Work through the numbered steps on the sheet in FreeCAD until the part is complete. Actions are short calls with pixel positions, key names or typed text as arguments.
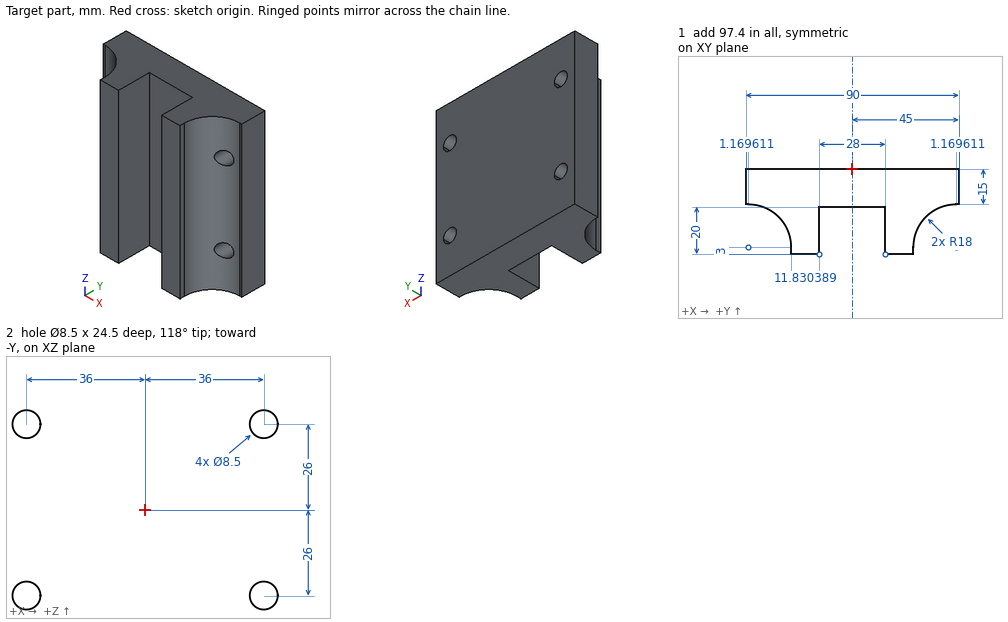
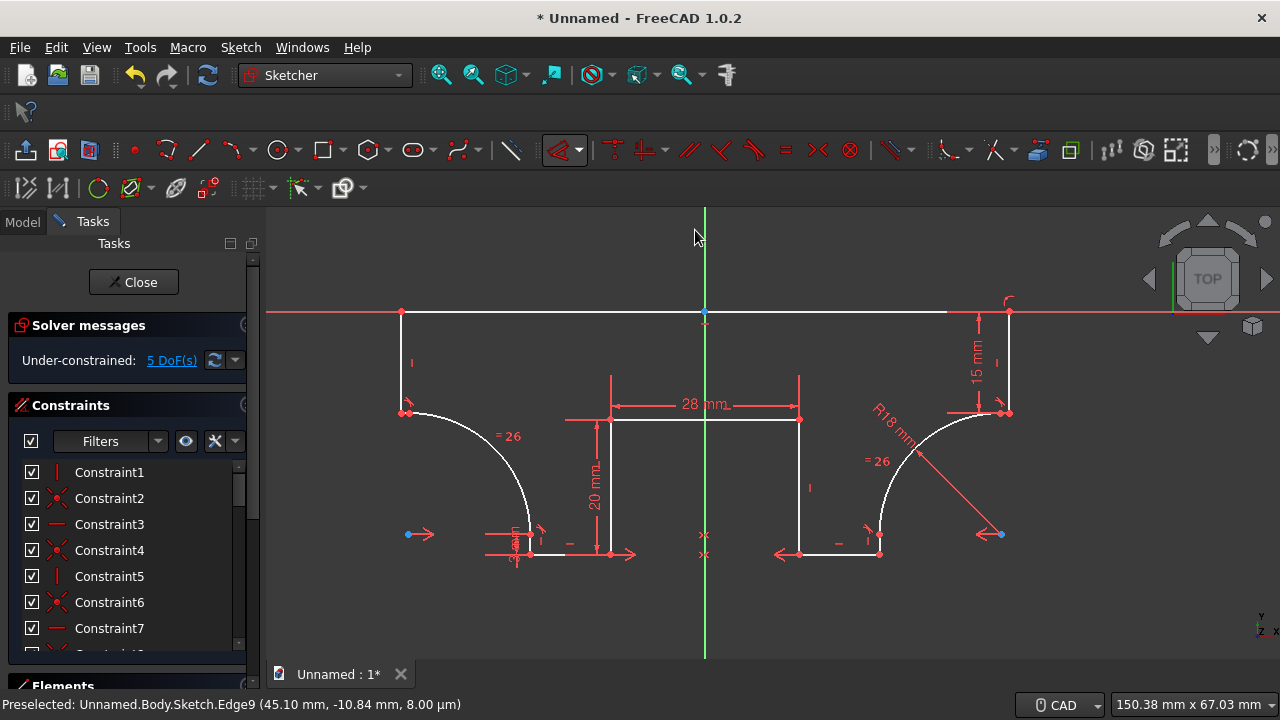
click(827, 312)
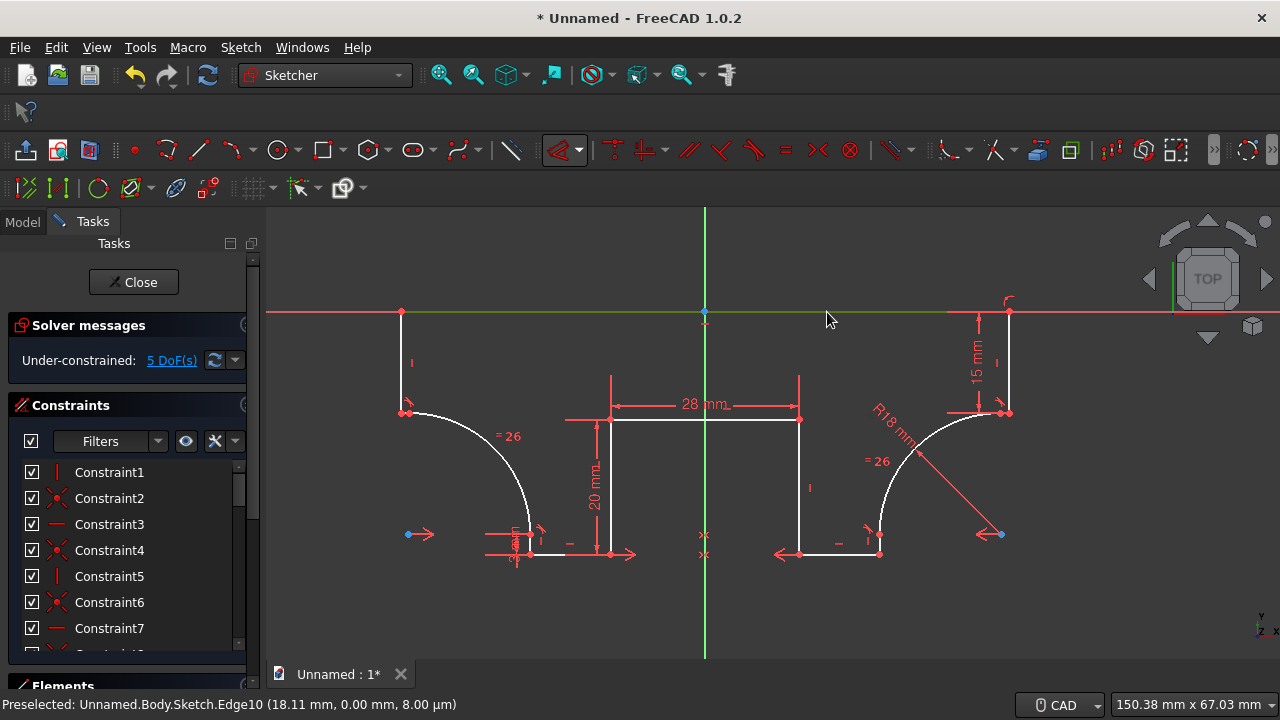
click(582, 150)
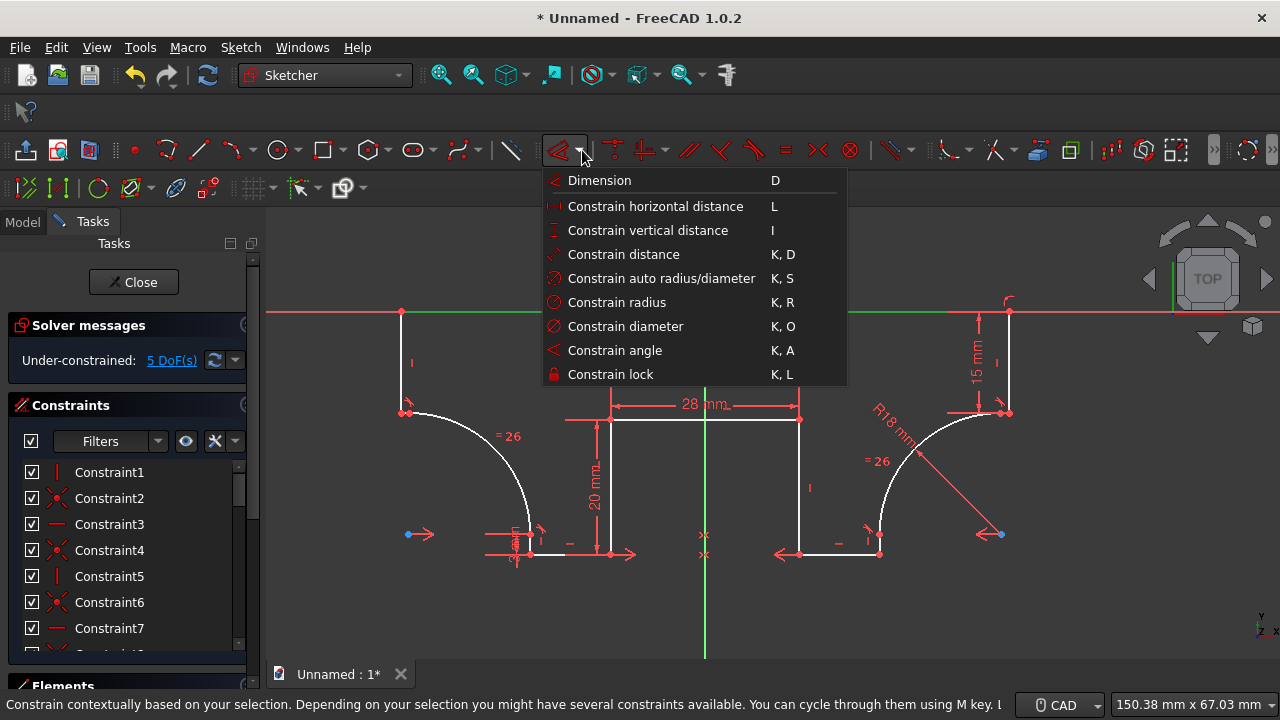
click(695, 206)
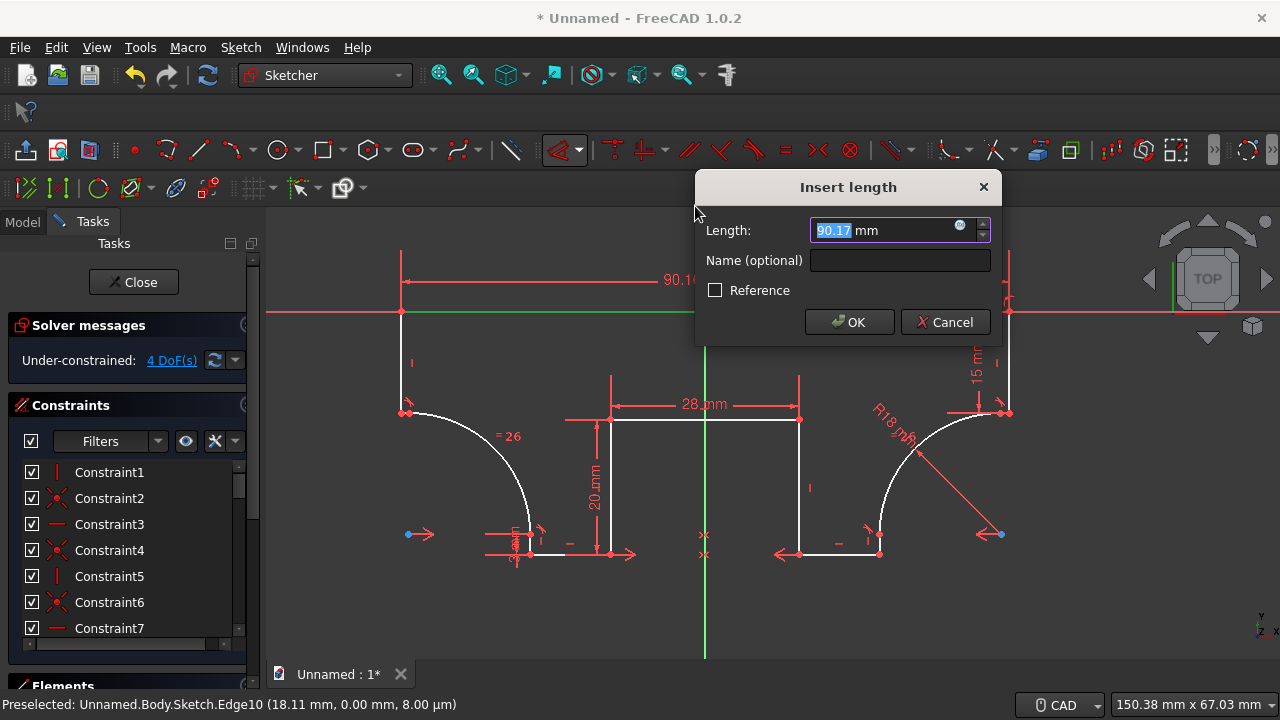
text(90)
key(Return)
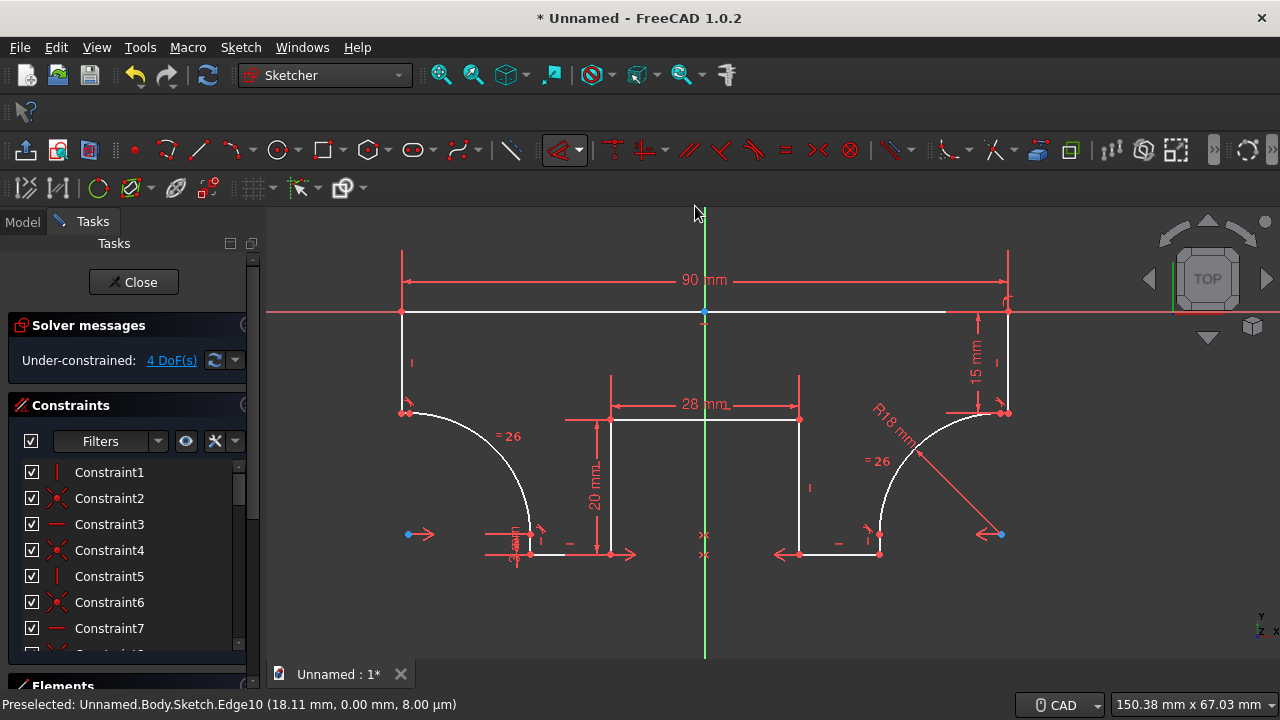
scroll(1008, 413, up, 3)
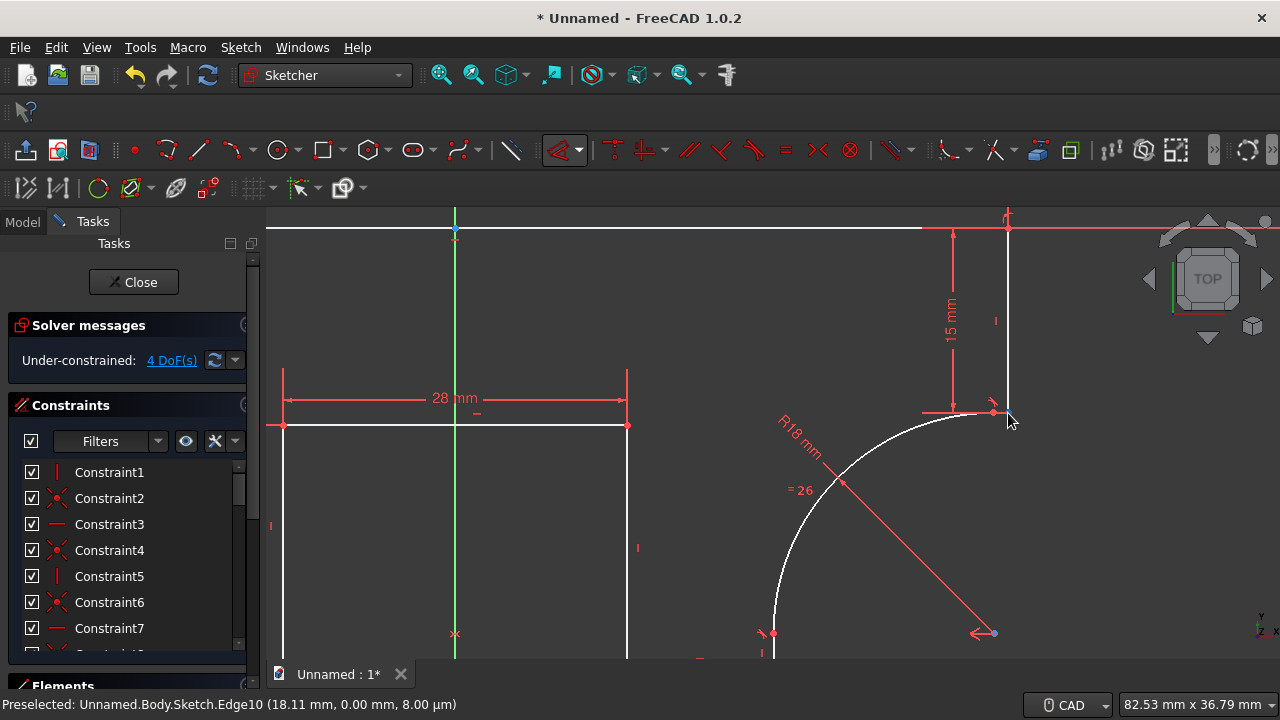
click(1008, 413)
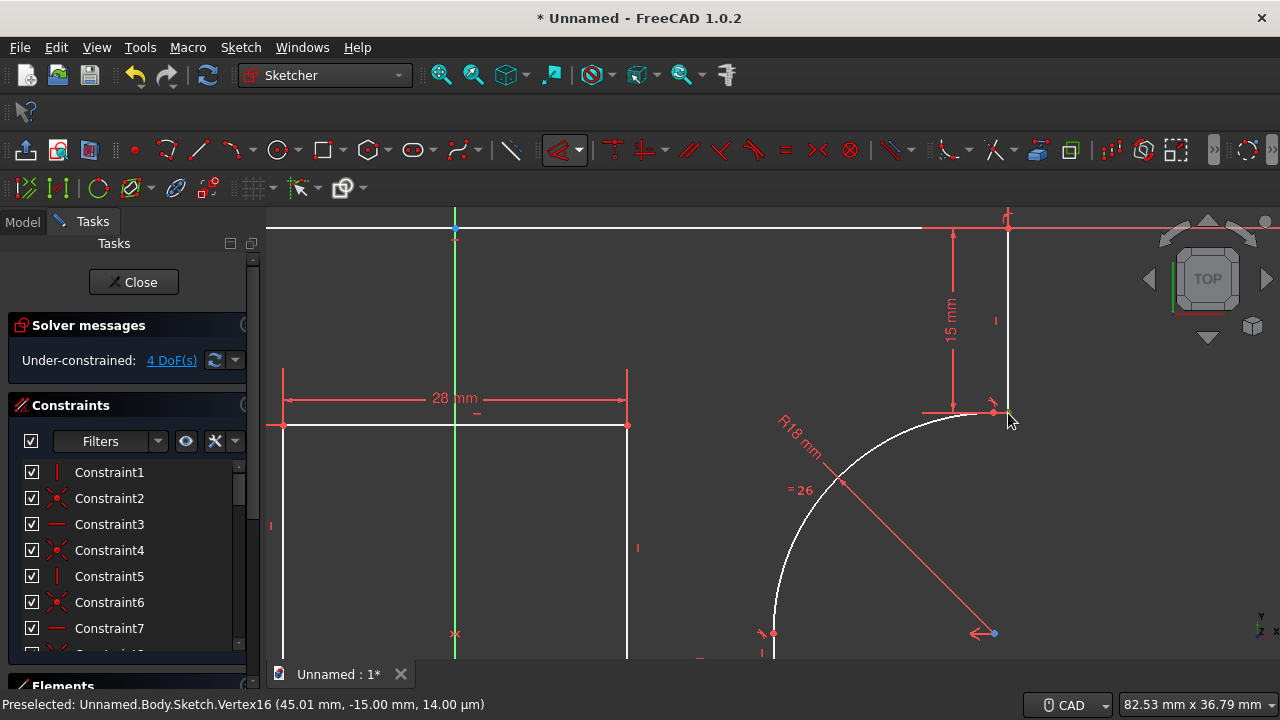
click(582, 150)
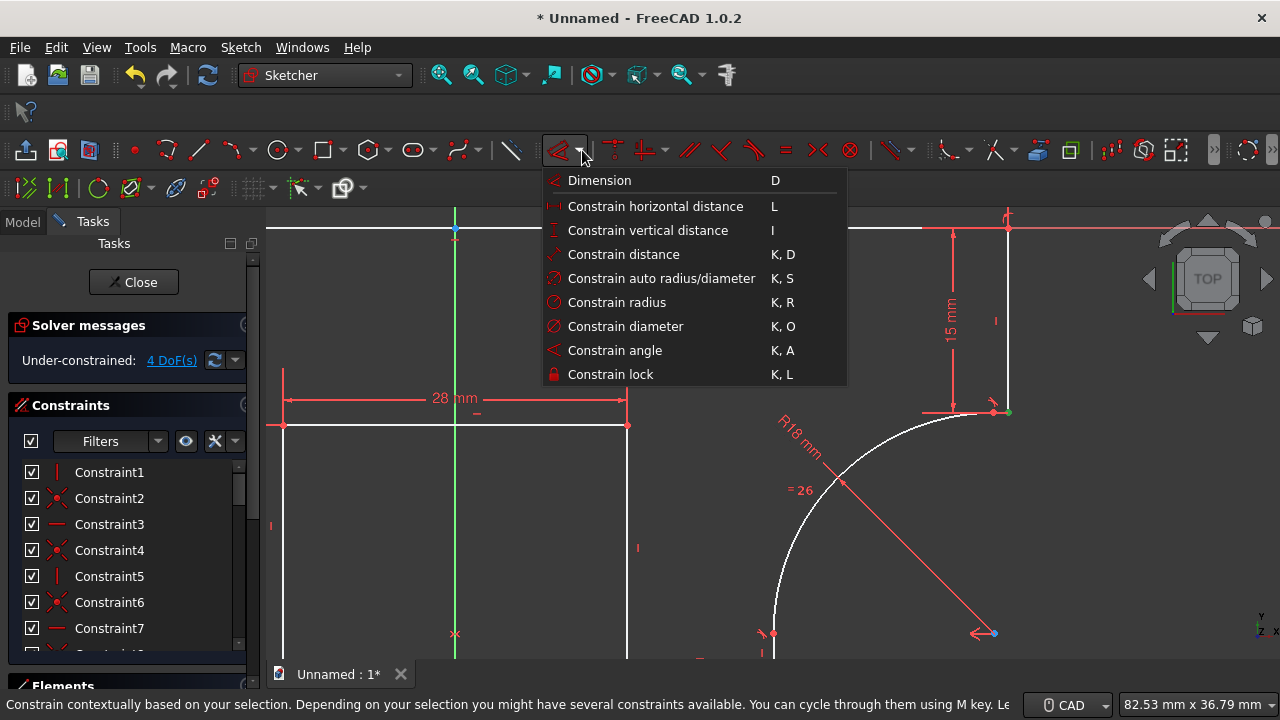
click(695, 206)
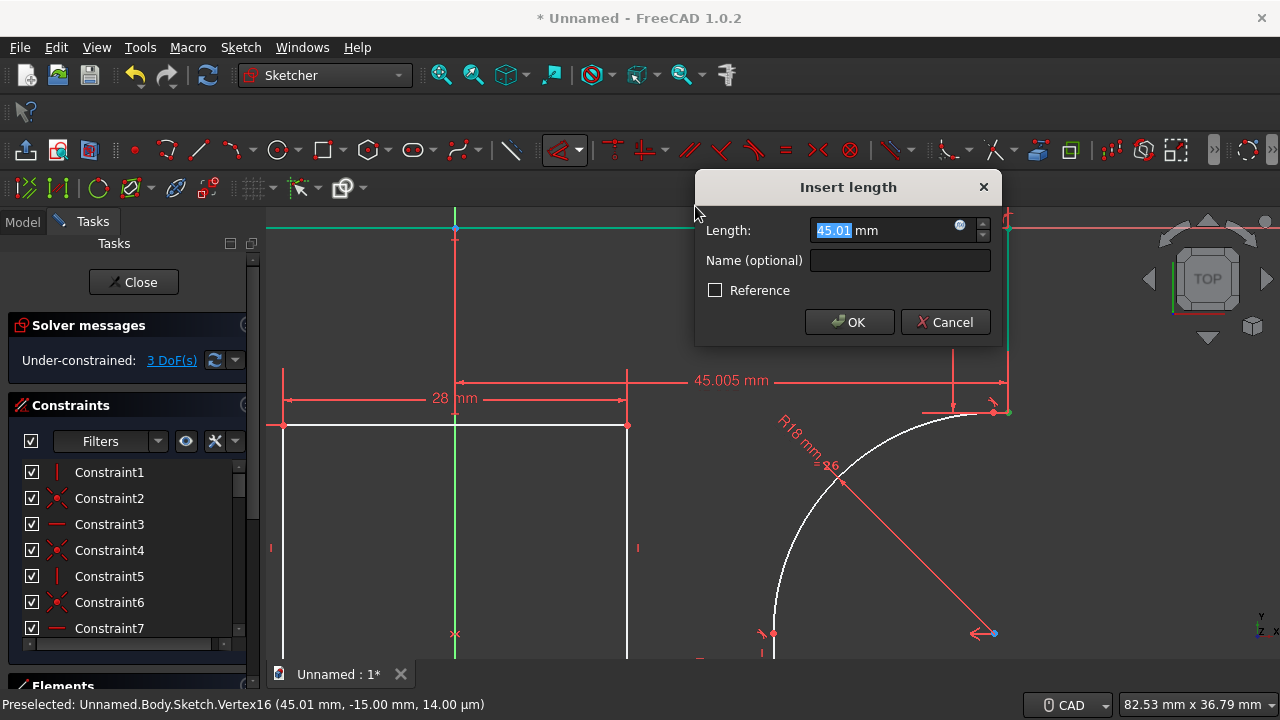
text(45)
key(Return)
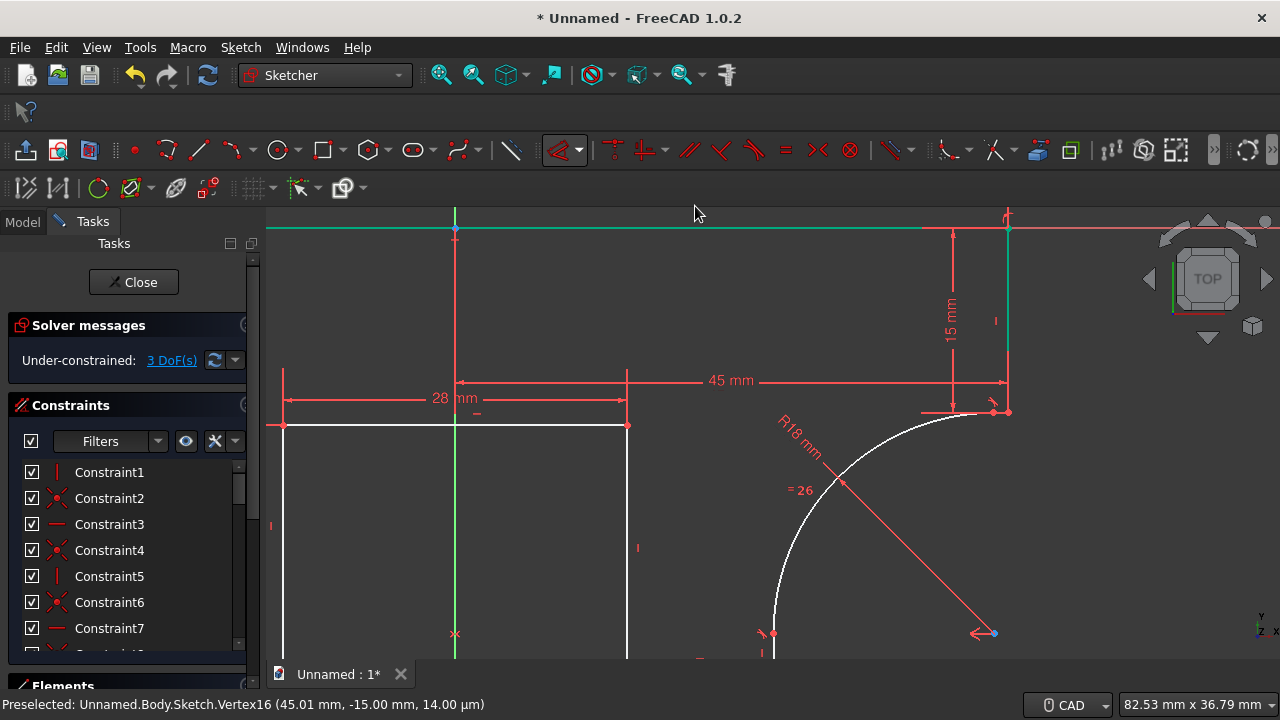
scroll(1001, 413, up, 6)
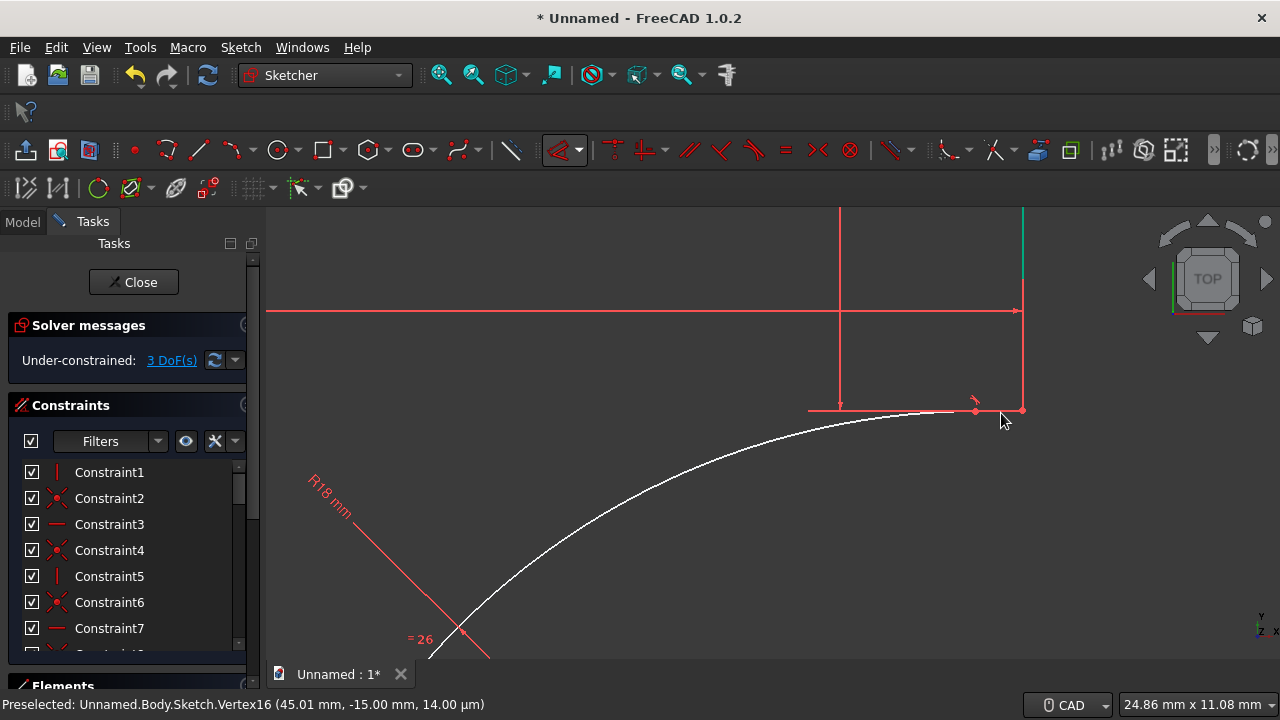
click(999, 411)